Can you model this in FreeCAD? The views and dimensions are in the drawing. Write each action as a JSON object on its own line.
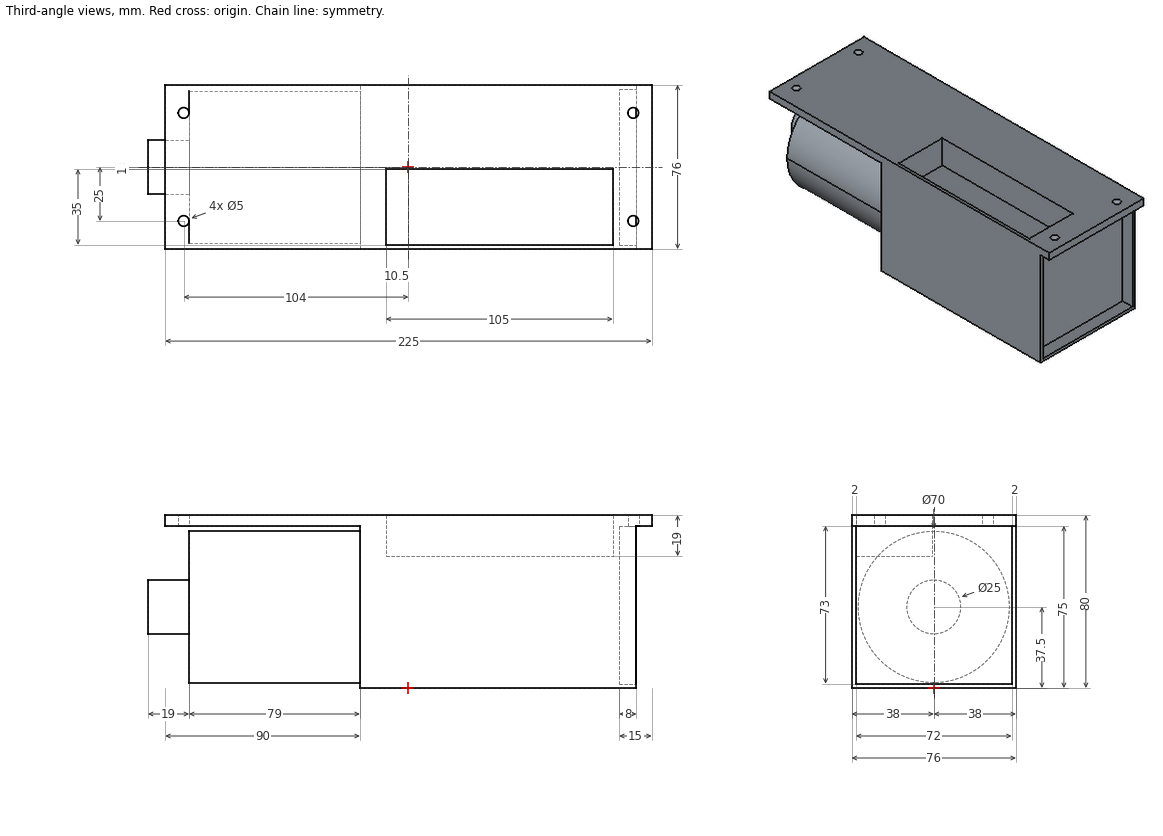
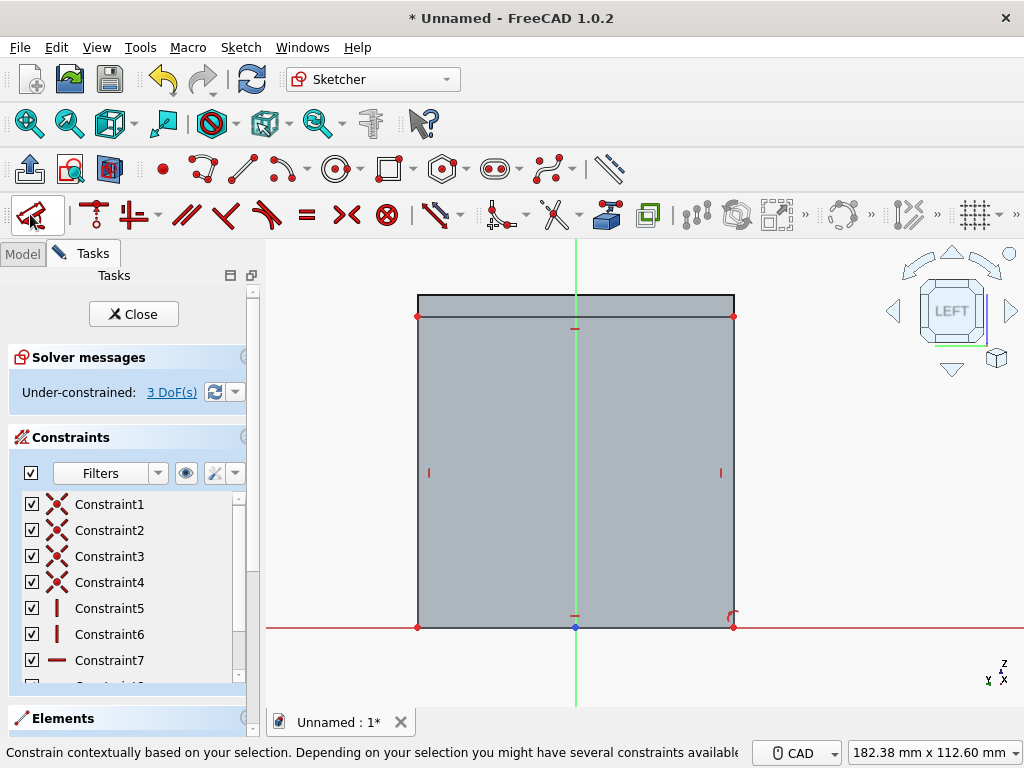
{"action": "left_click", "coordinate": [418, 410]}
{"action": "left_click", "coordinate": [384, 472]}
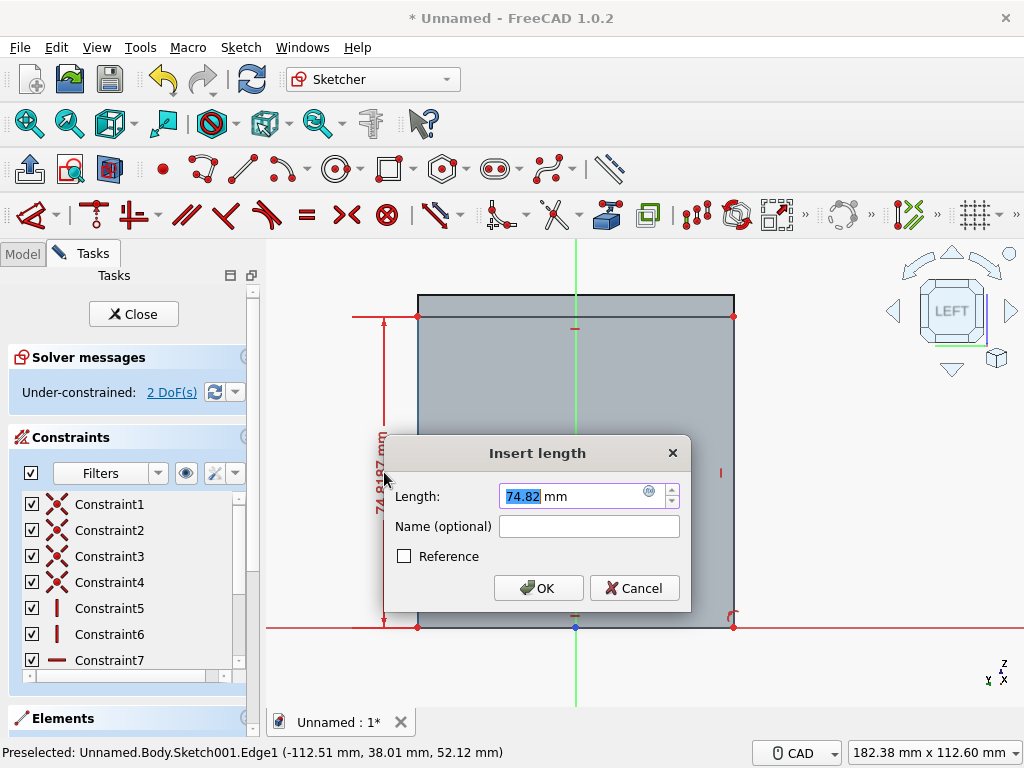
{"action": "type", "text": "75"}
{"action": "key", "text": "Return"}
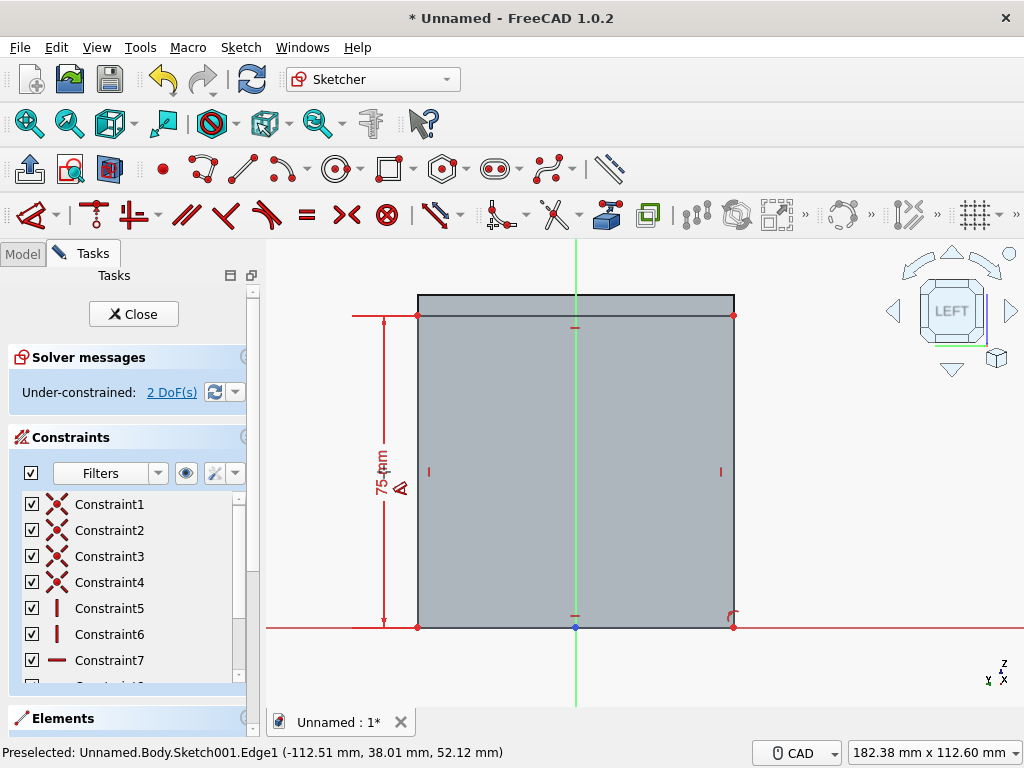
{"action": "left_click", "coordinate": [513, 628]}
{"action": "left_click", "coordinate": [503, 662]}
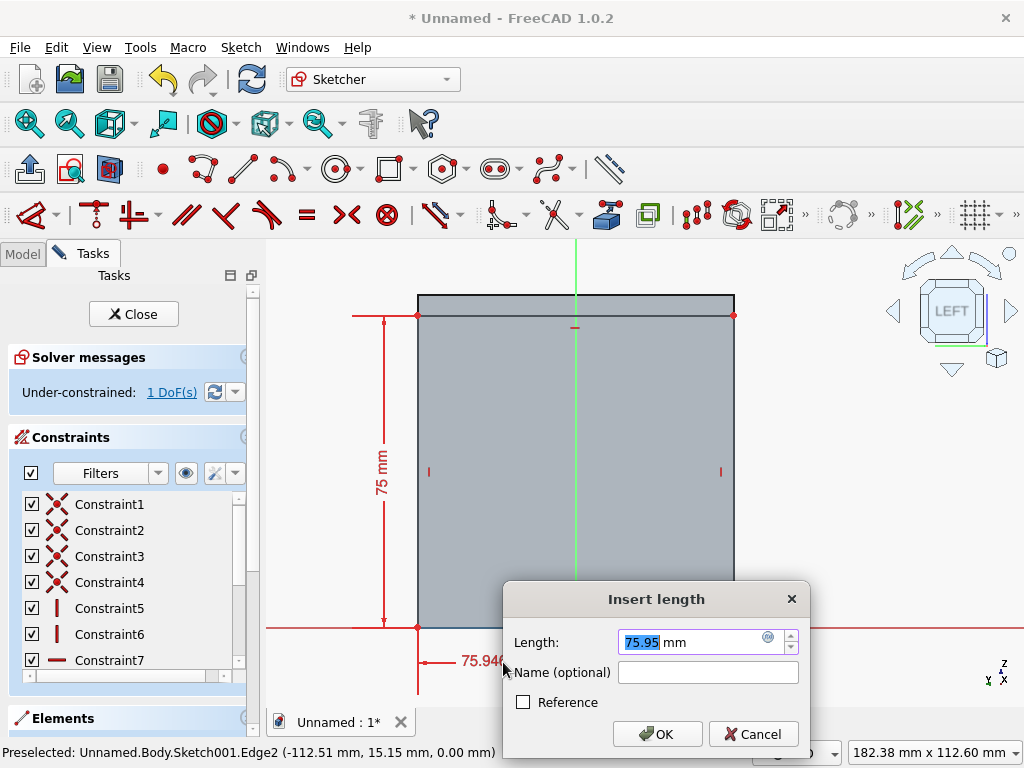
{"action": "type", "text": "76"}
{"action": "key", "text": "Return"}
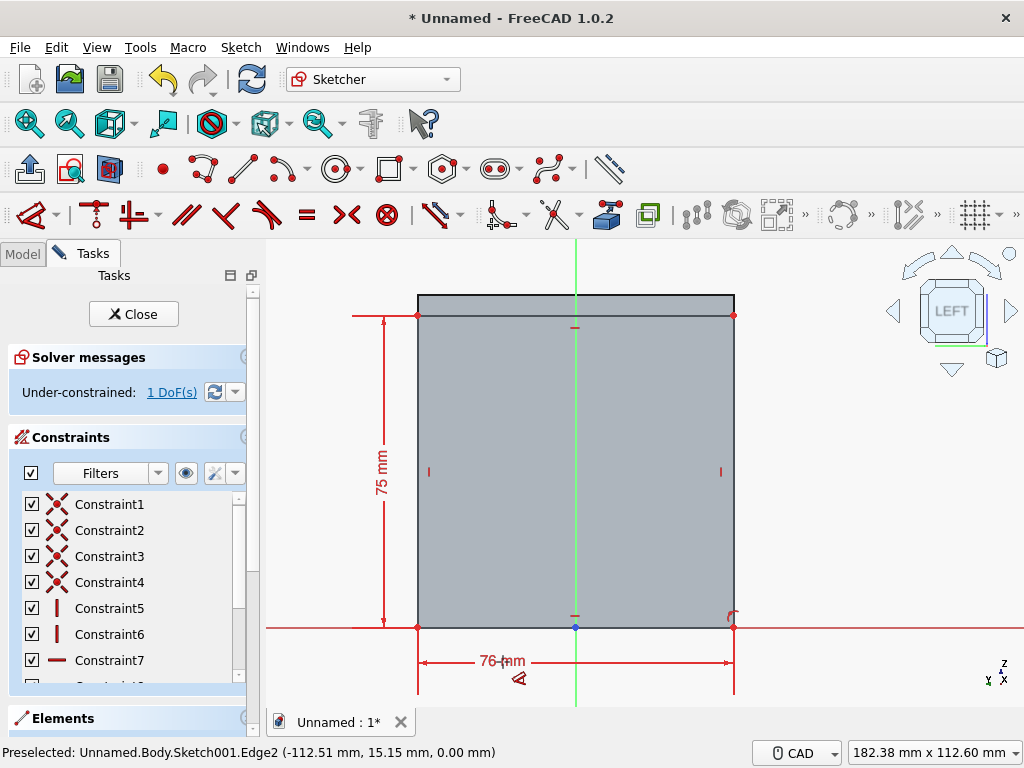
{"action": "left_click", "coordinate": [418, 316]}
{"action": "left_click", "coordinate": [497, 282]}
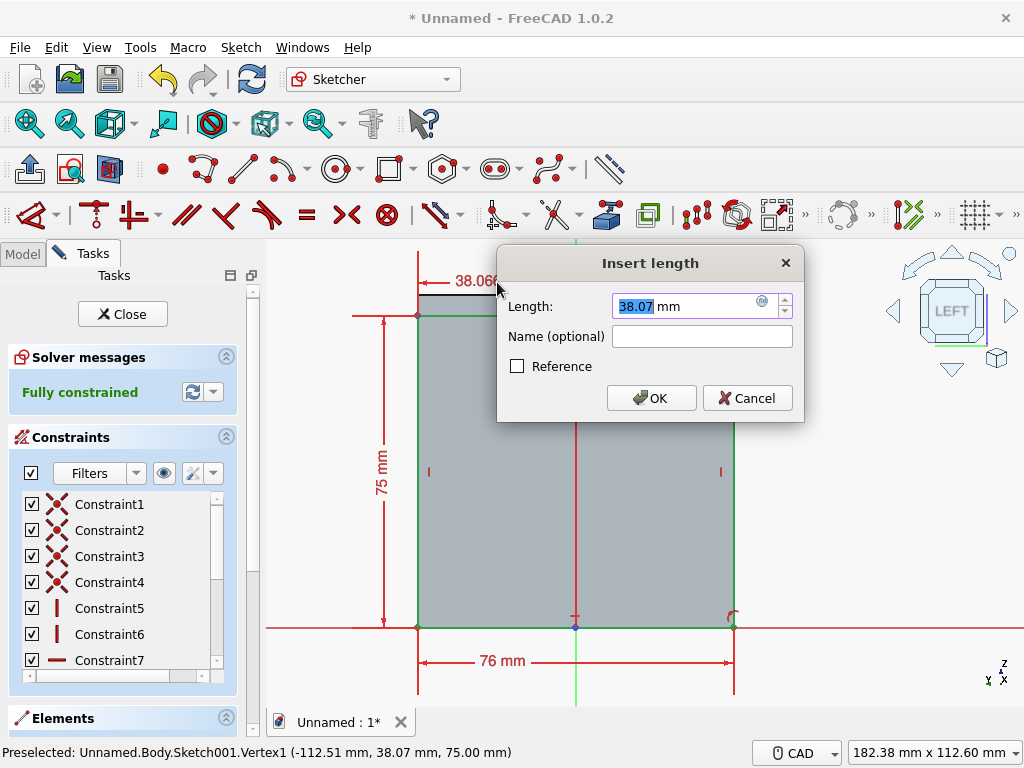
{"action": "type", "text": "38"}
{"action": "key", "text": "Return"}
{"action": "key", "text": "Escape"}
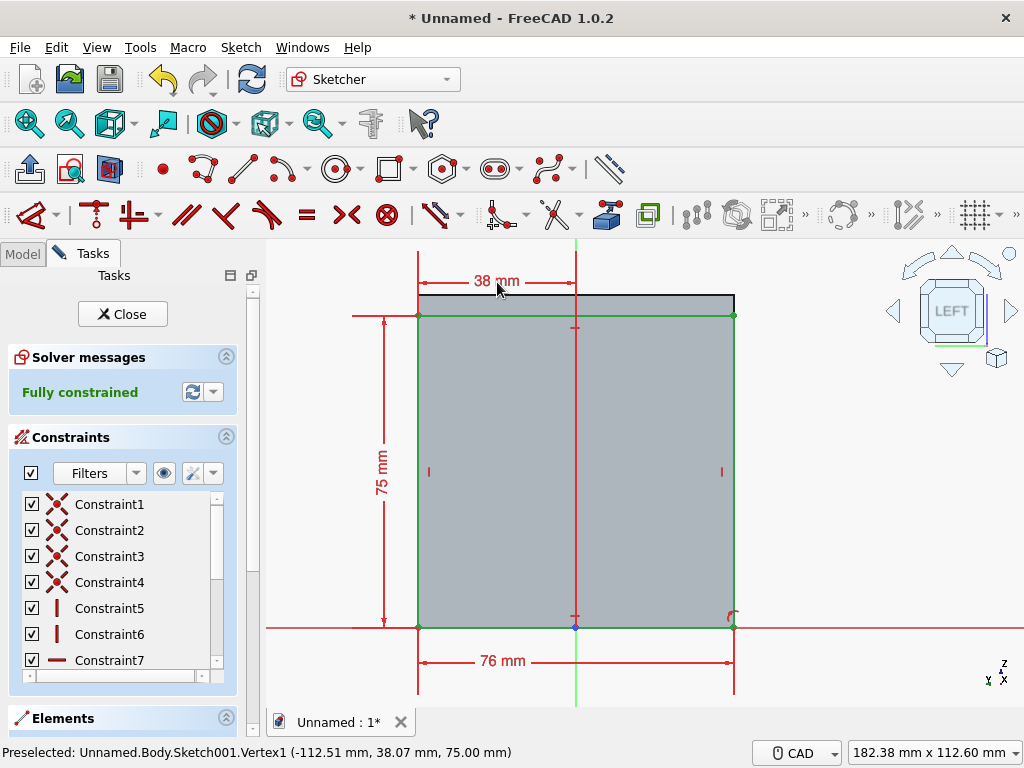
{"action": "left_click", "coordinate": [123, 314]}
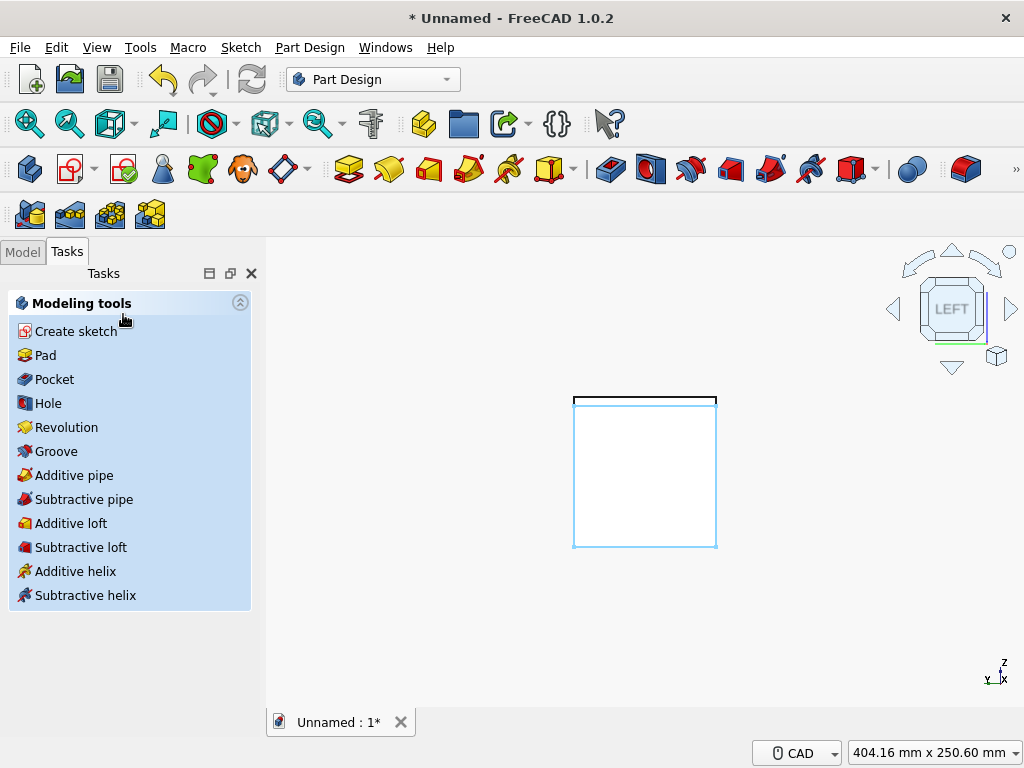
{"action": "left_click", "coordinate": [612, 170]}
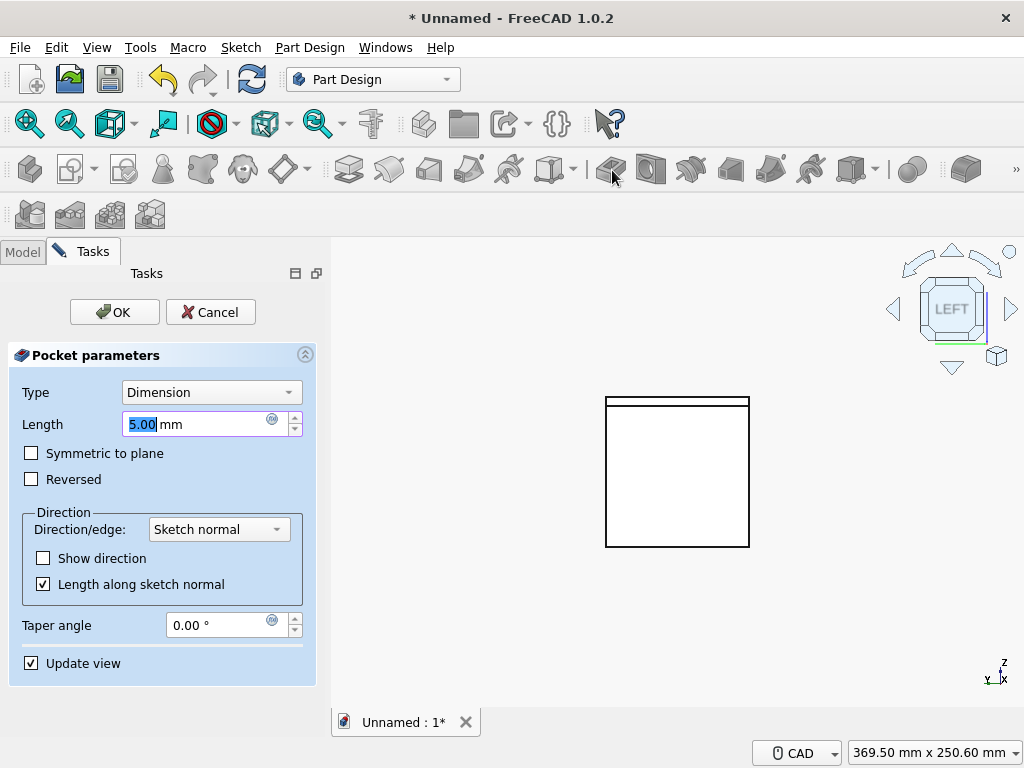
{"action": "type", "text": "90"}
{"action": "key", "text": "Tab"}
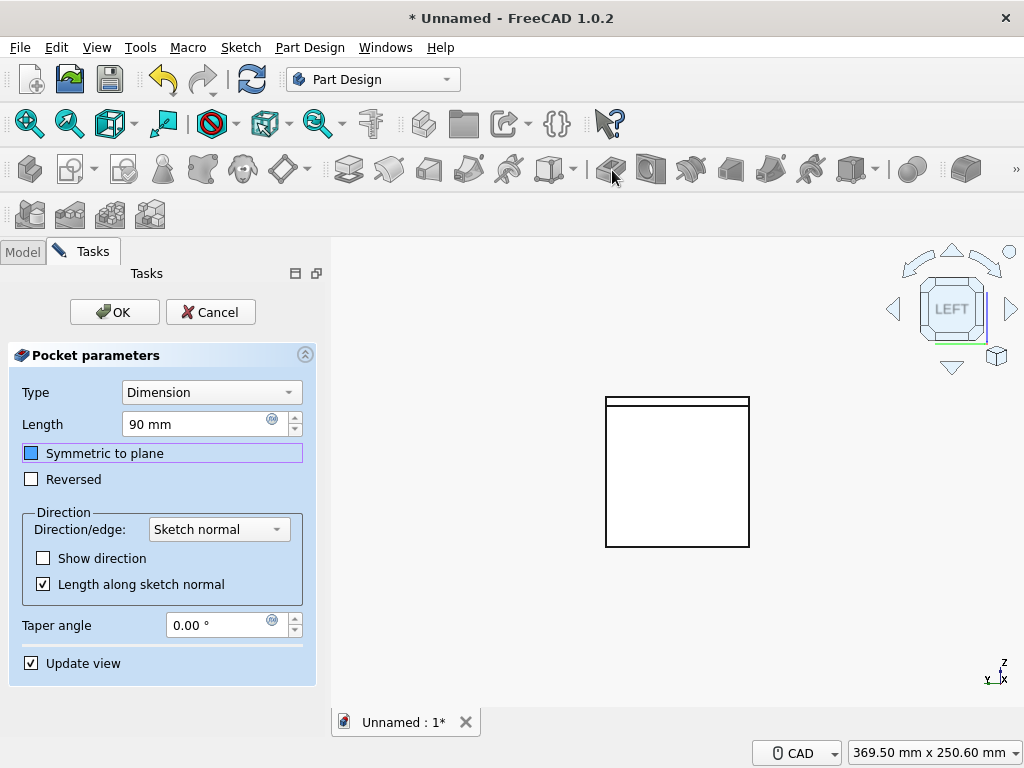
{"action": "left_click", "coordinate": [115, 312]}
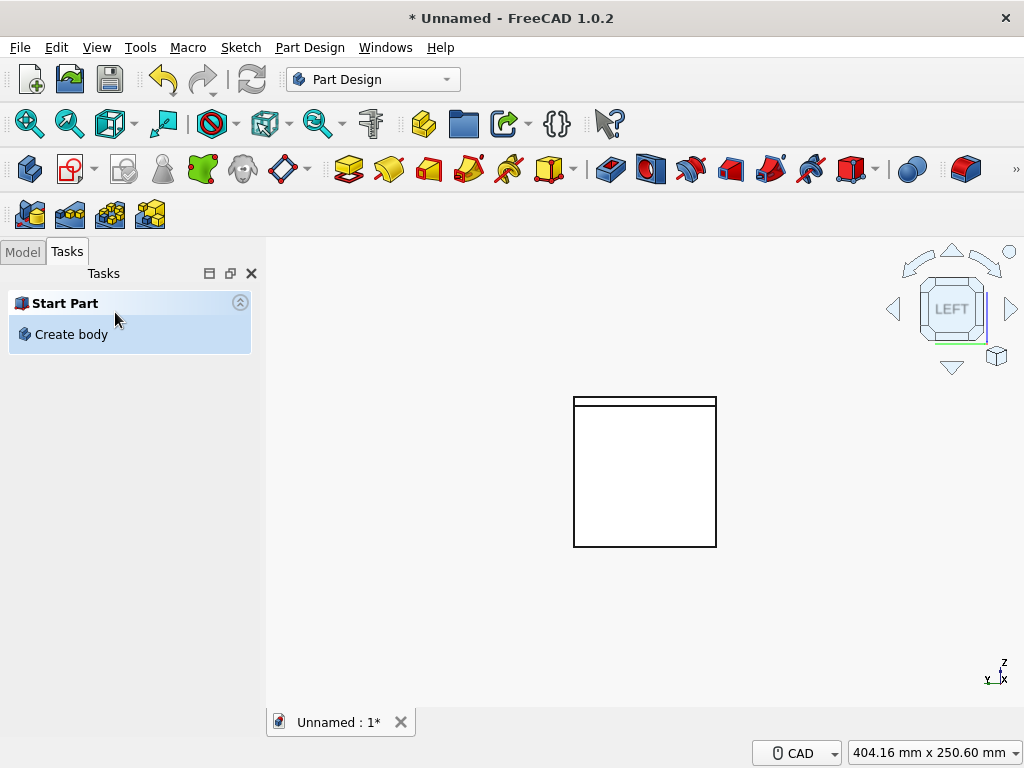
{"action": "left_click", "coordinate": [30, 124]}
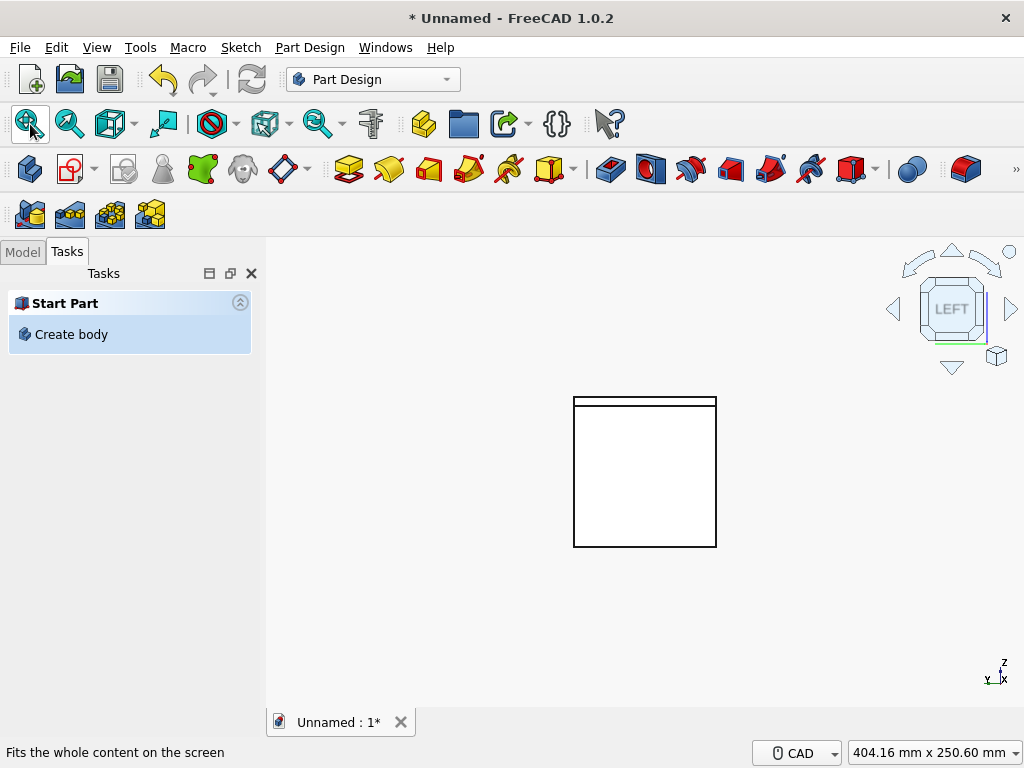
{"action": "key", "text": "0"}